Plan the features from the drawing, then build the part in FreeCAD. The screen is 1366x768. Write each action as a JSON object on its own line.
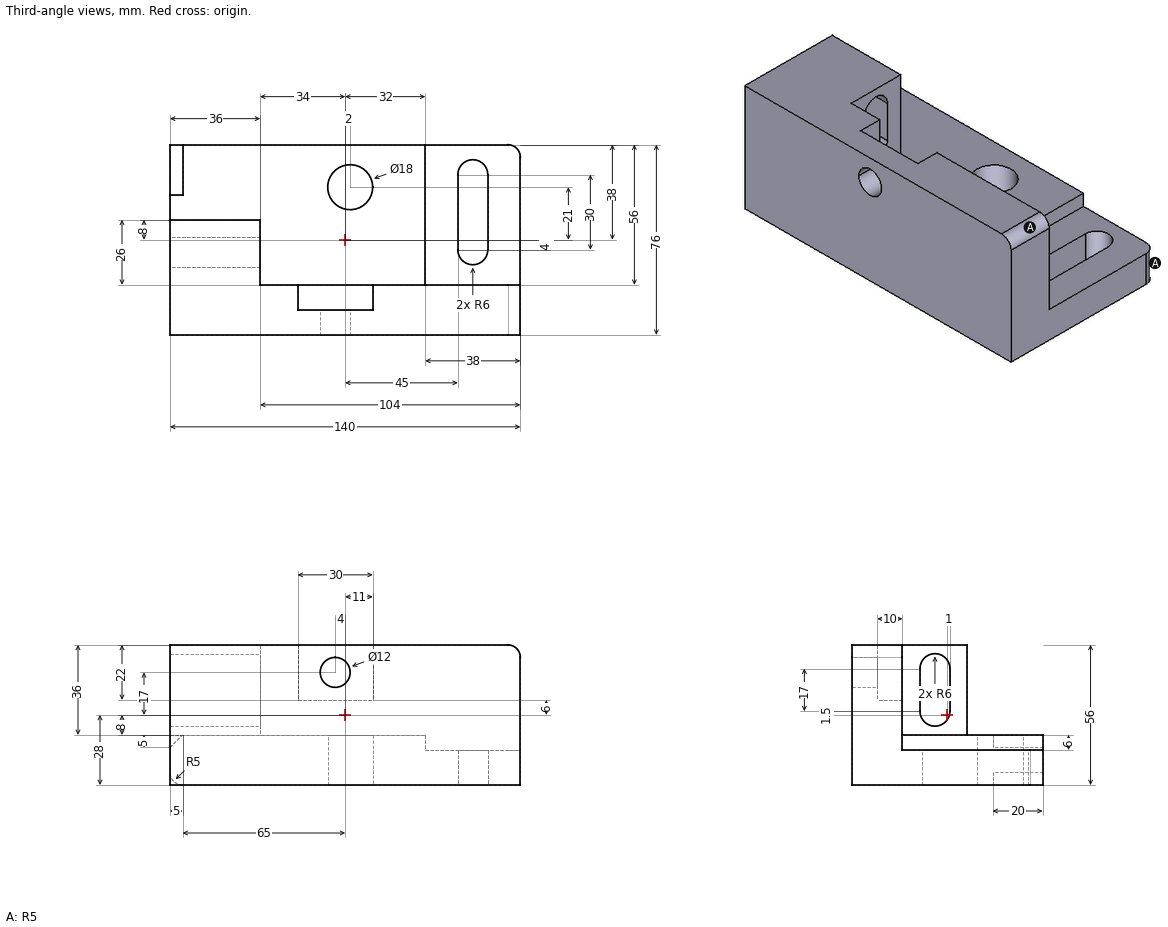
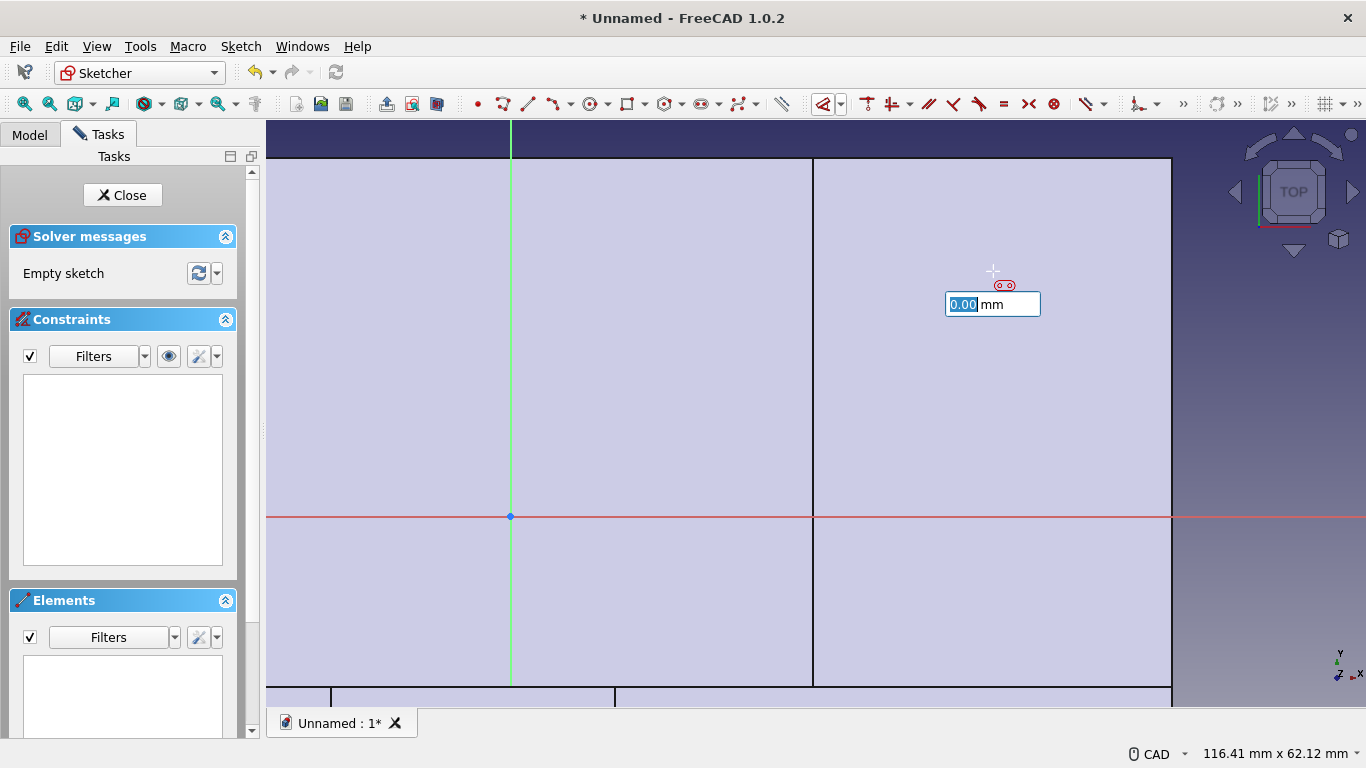
{"action": "left_click", "coordinate": [936, 413]}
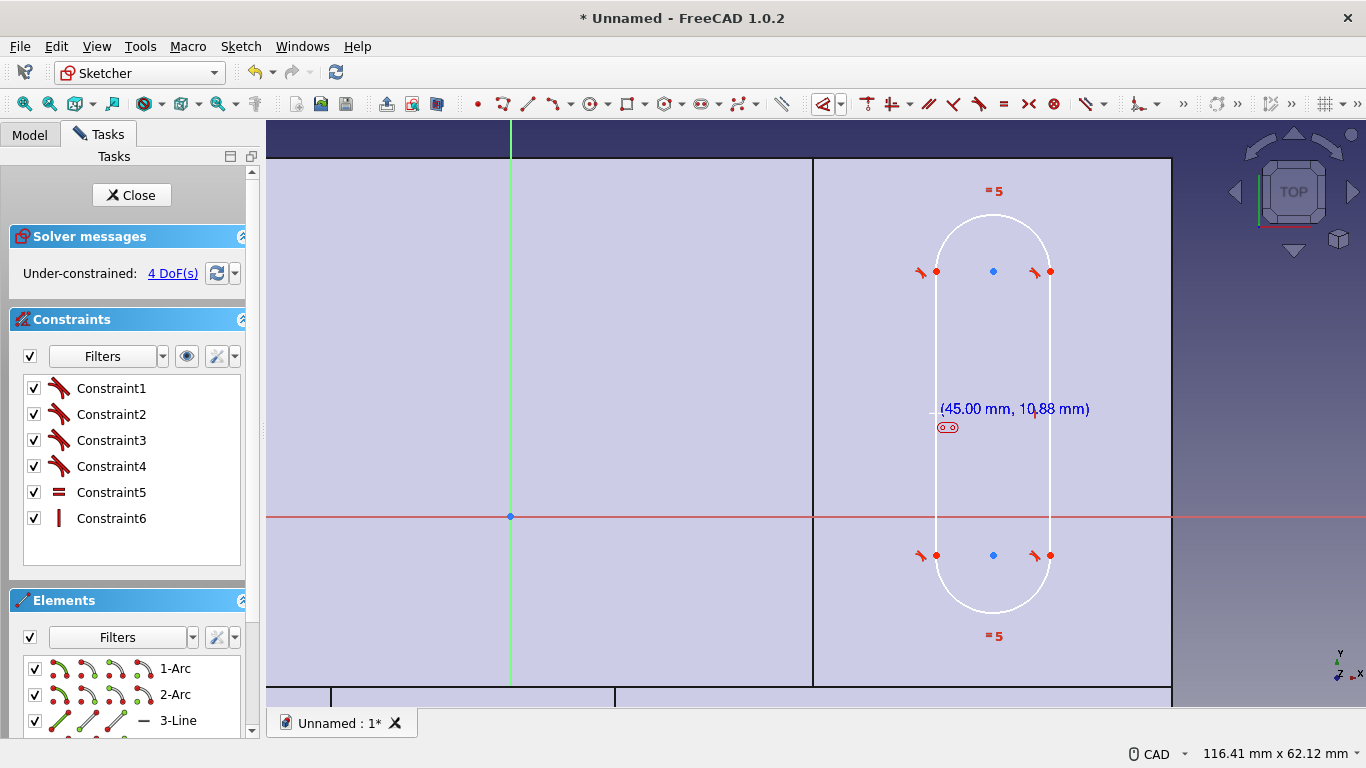
{"action": "left_click", "coordinate": [590, 104]}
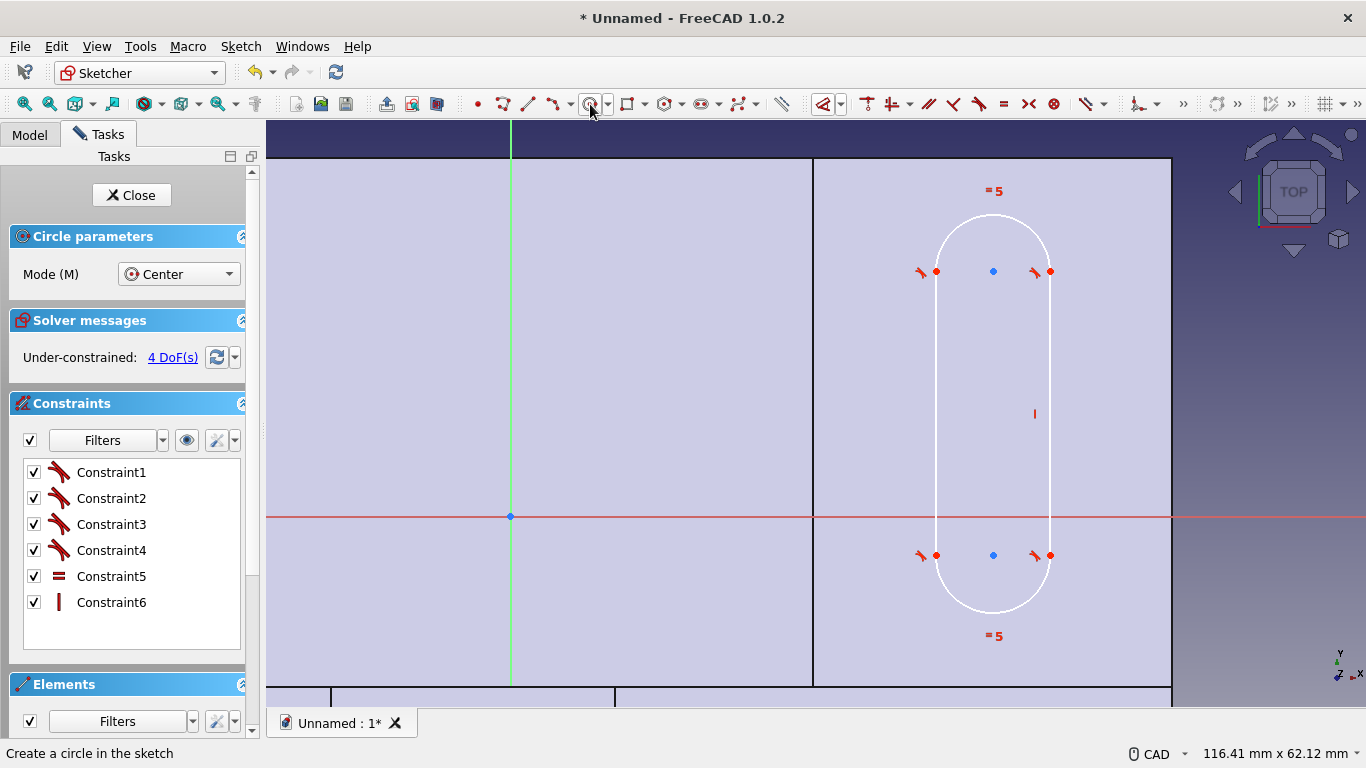
{"action": "left_click", "coordinate": [530, 318]}
{"action": "mouse_move", "coordinate": [590, 258]}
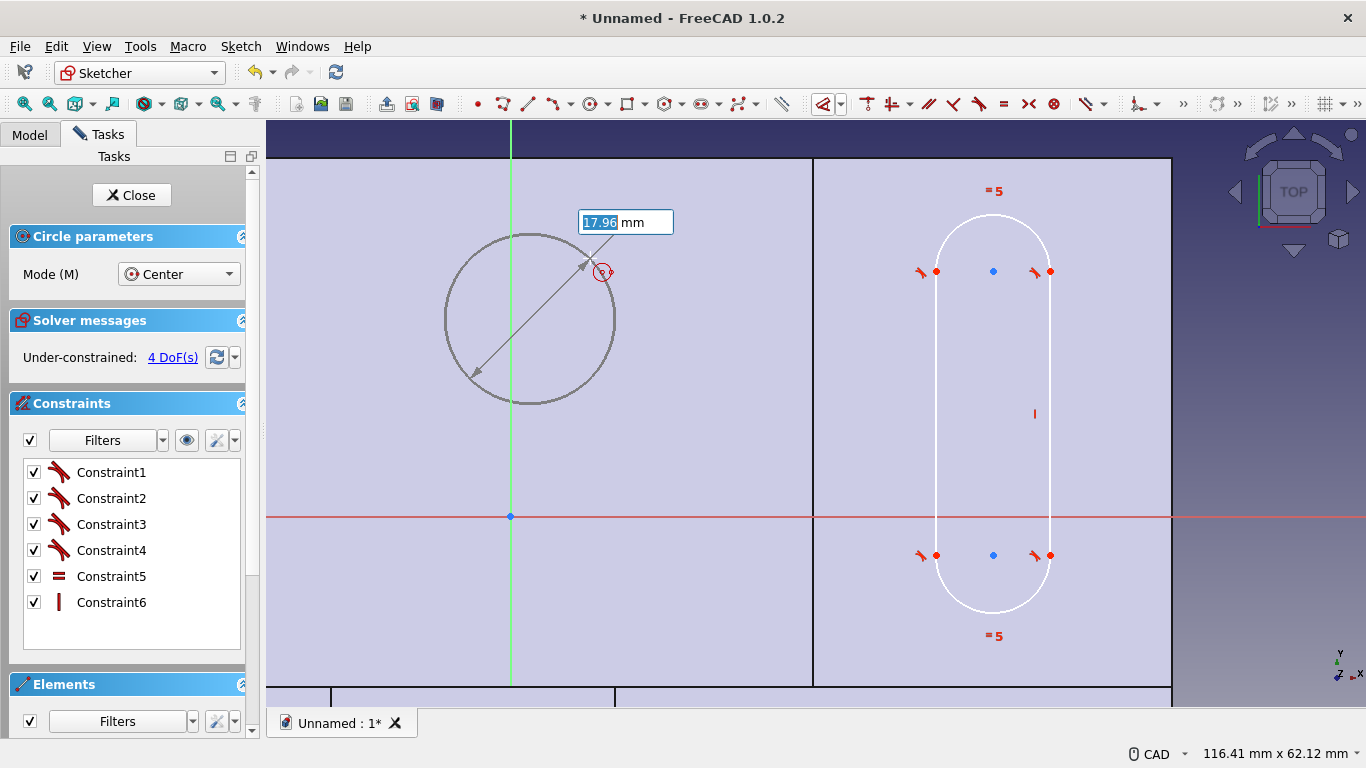
{"action": "type", "text": "18"}
{"action": "key", "text": "Return"}
{"action": "key", "text": "Escape"}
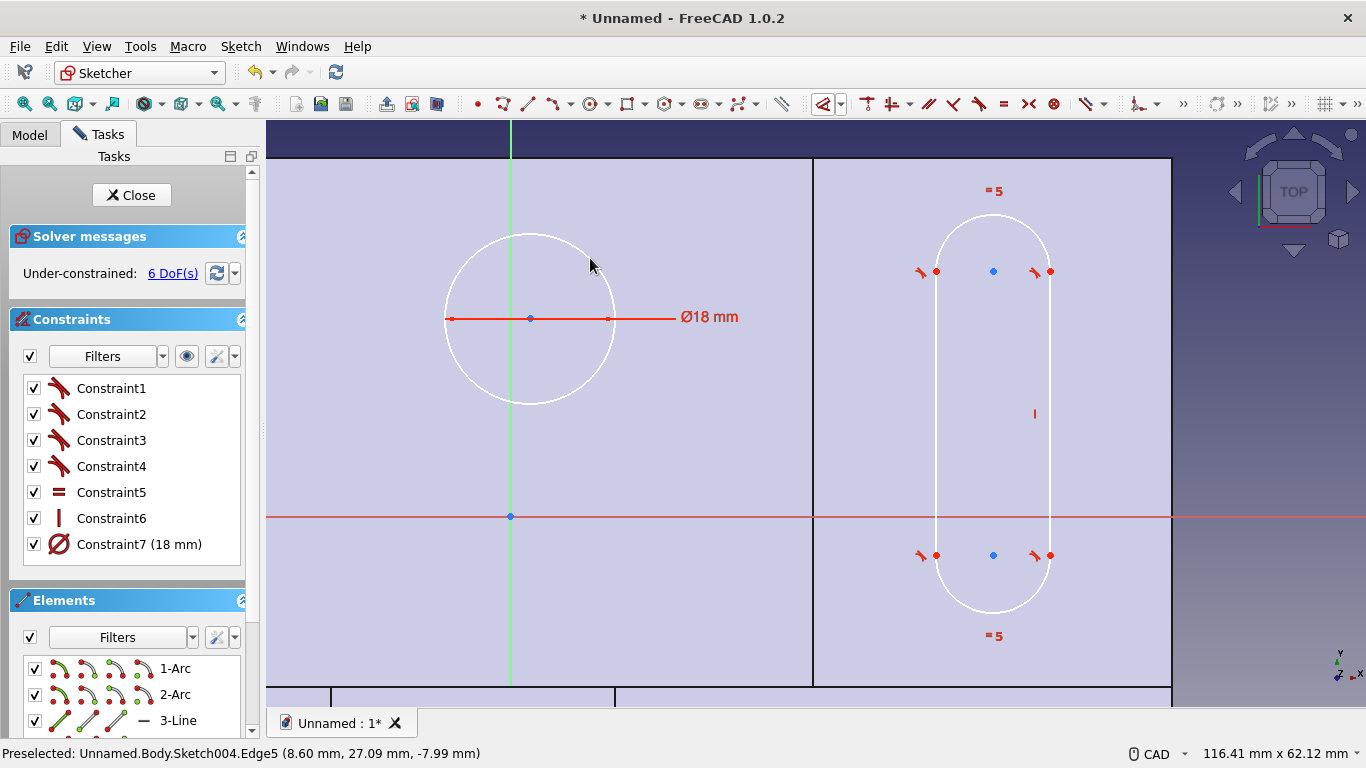
{"action": "left_click", "coordinate": [959, 602]}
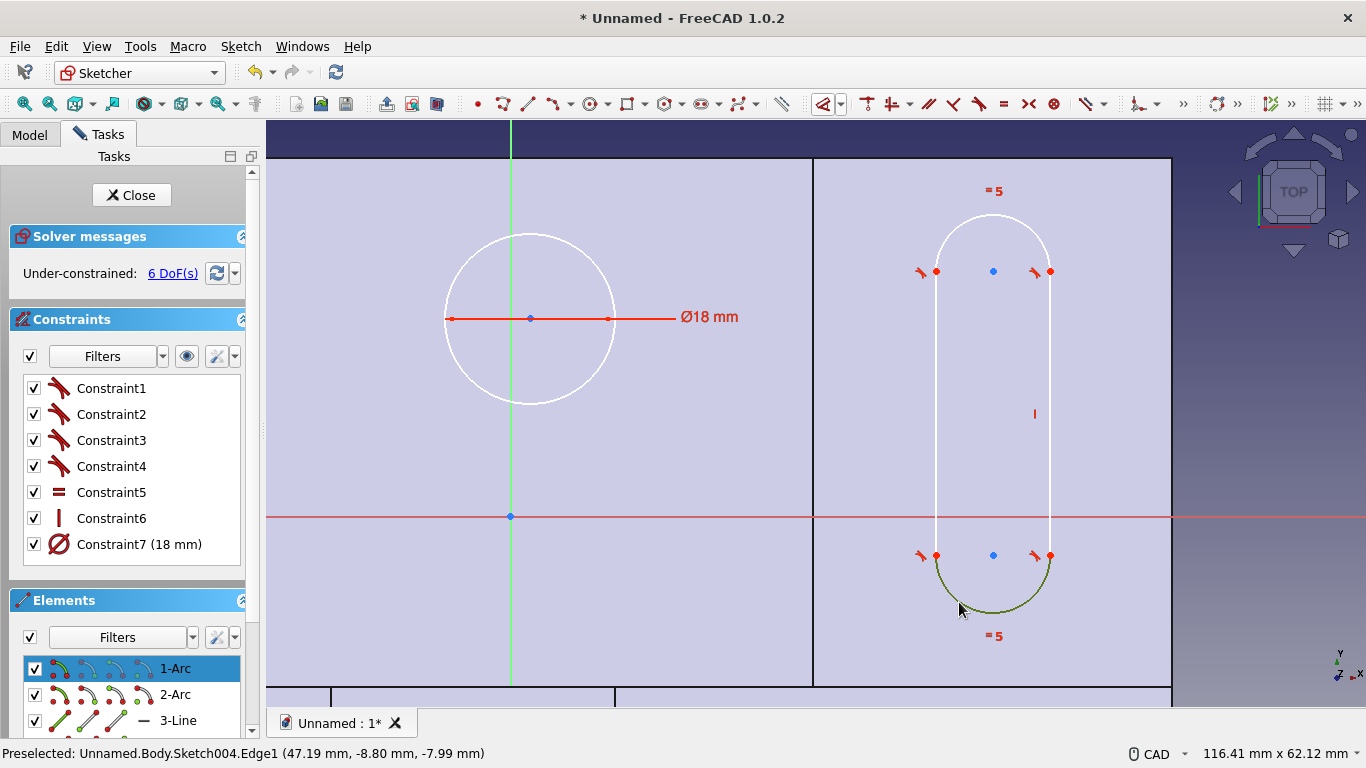
{"action": "key", "text": "k r"}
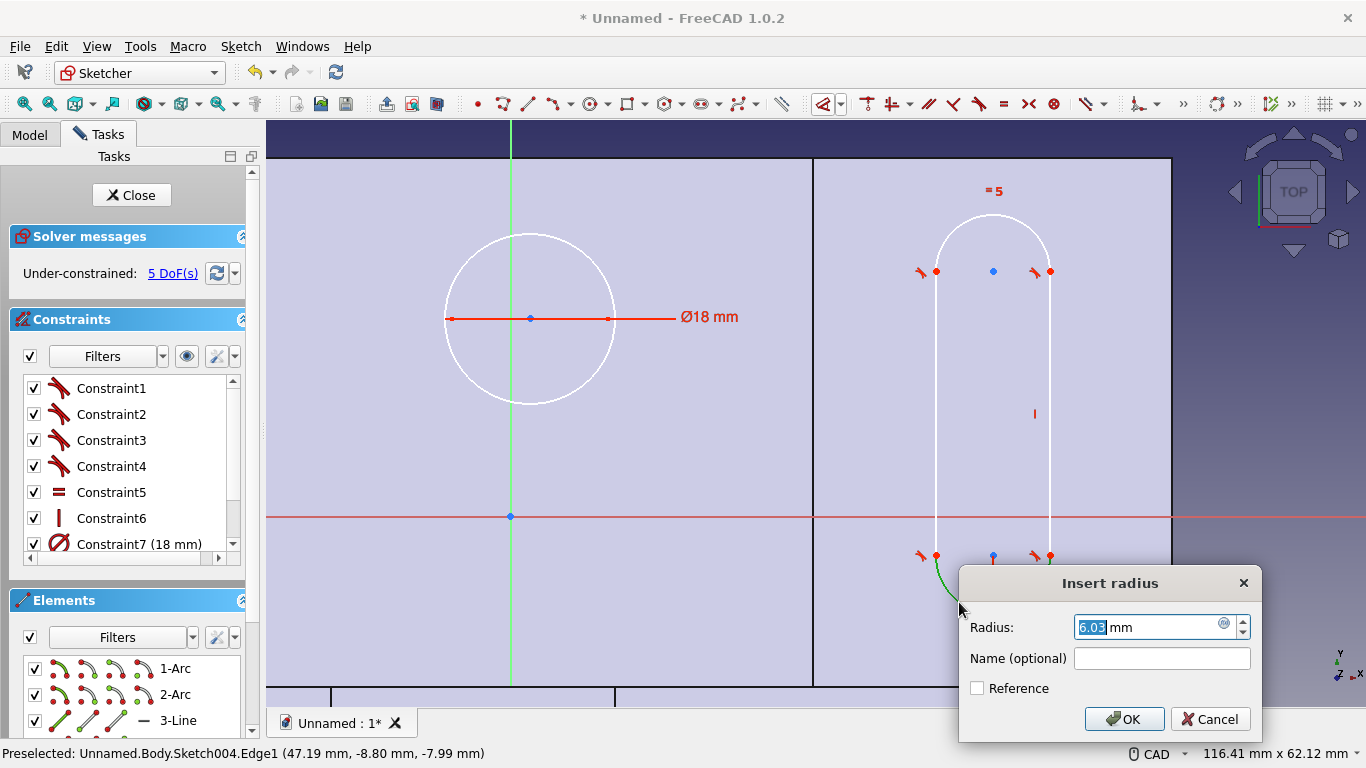
{"action": "type", "text": "6"}
{"action": "key", "text": "Return"}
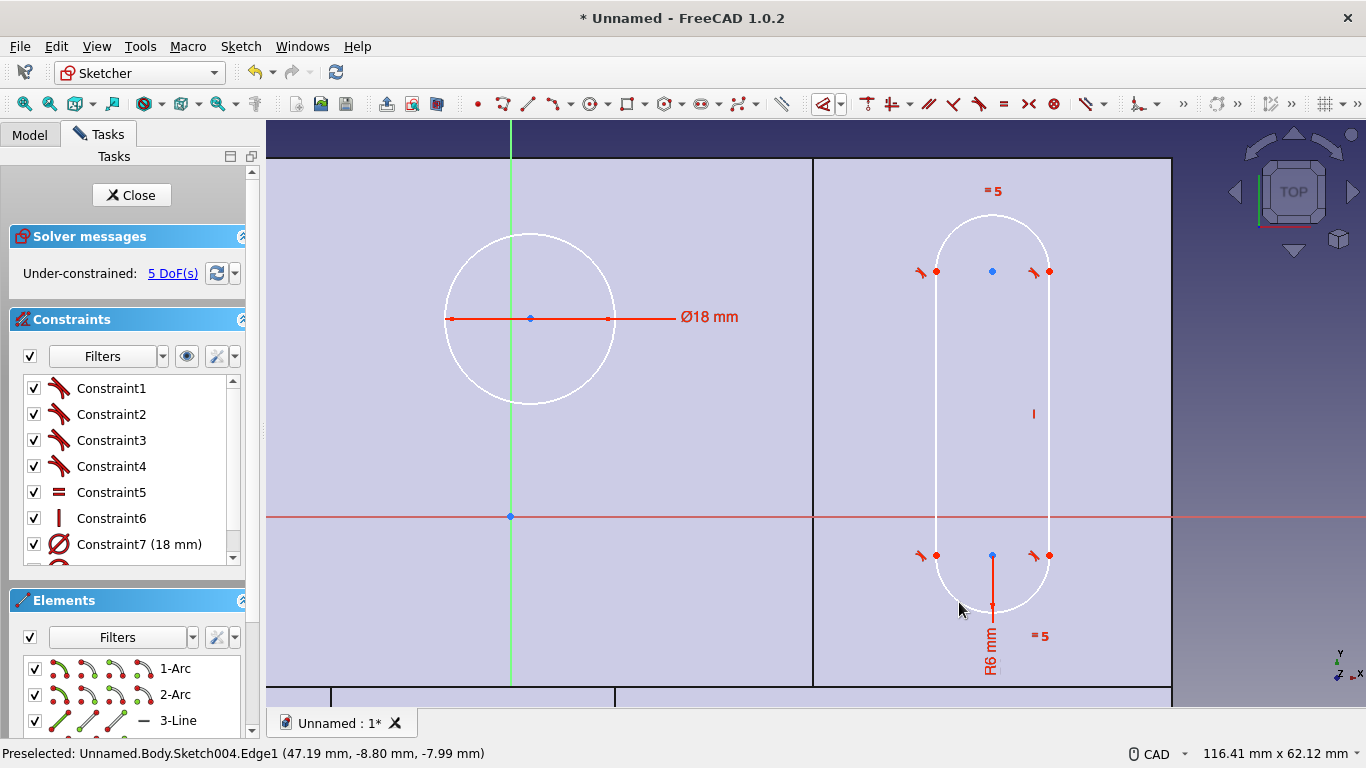
{"action": "scroll", "coordinate": [530, 319], "scroll_direction": "up", "scroll_amount": 4}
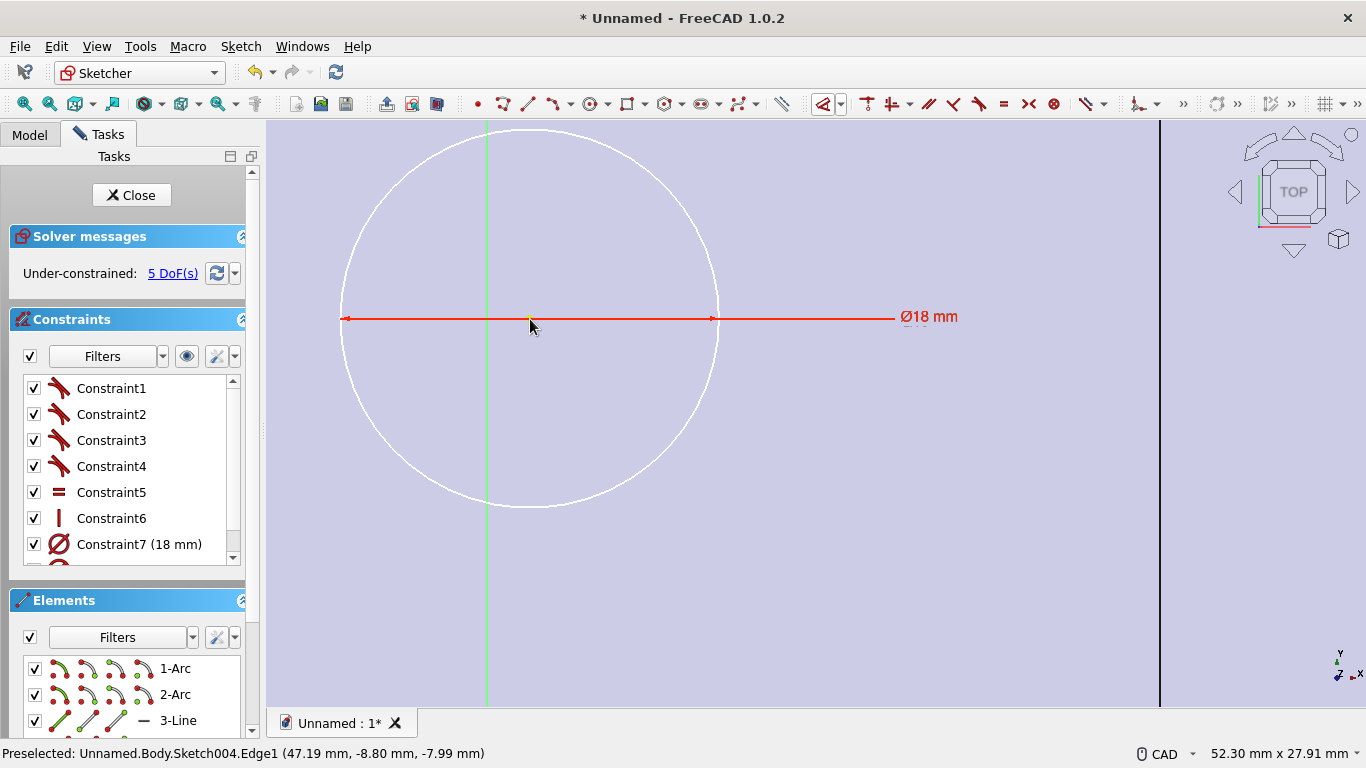
{"action": "left_click", "coordinate": [530, 319]}